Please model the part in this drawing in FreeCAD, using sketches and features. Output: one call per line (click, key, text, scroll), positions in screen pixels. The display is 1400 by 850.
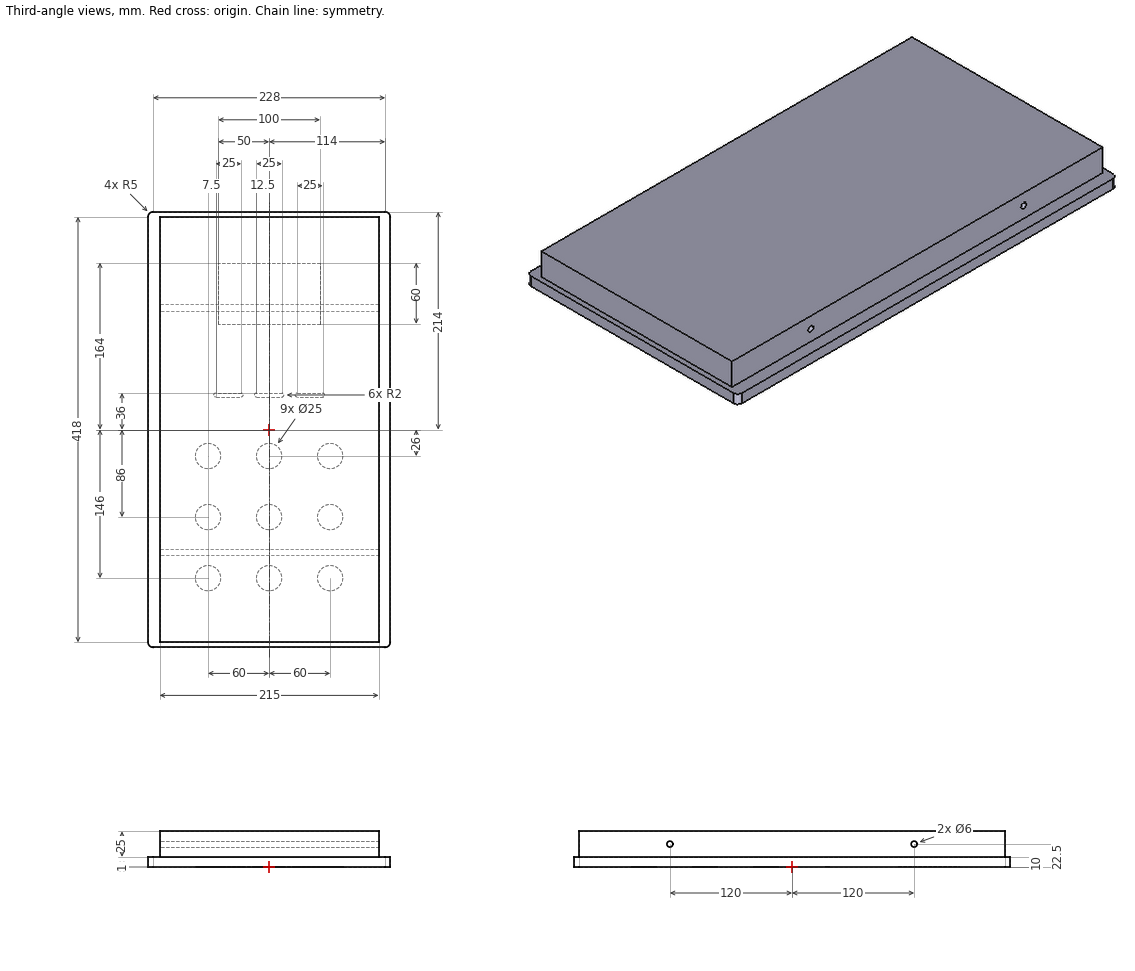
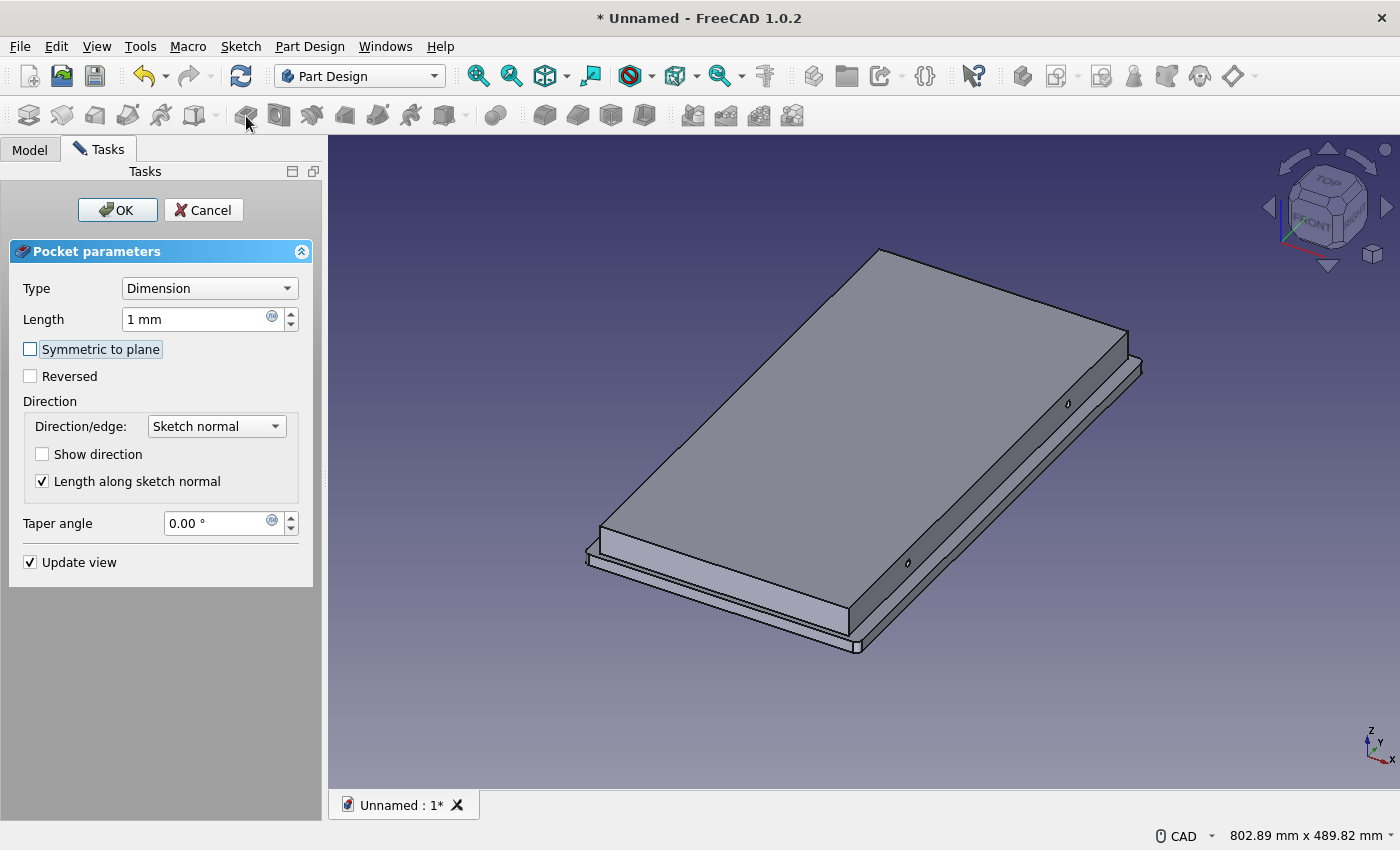
click(31, 376)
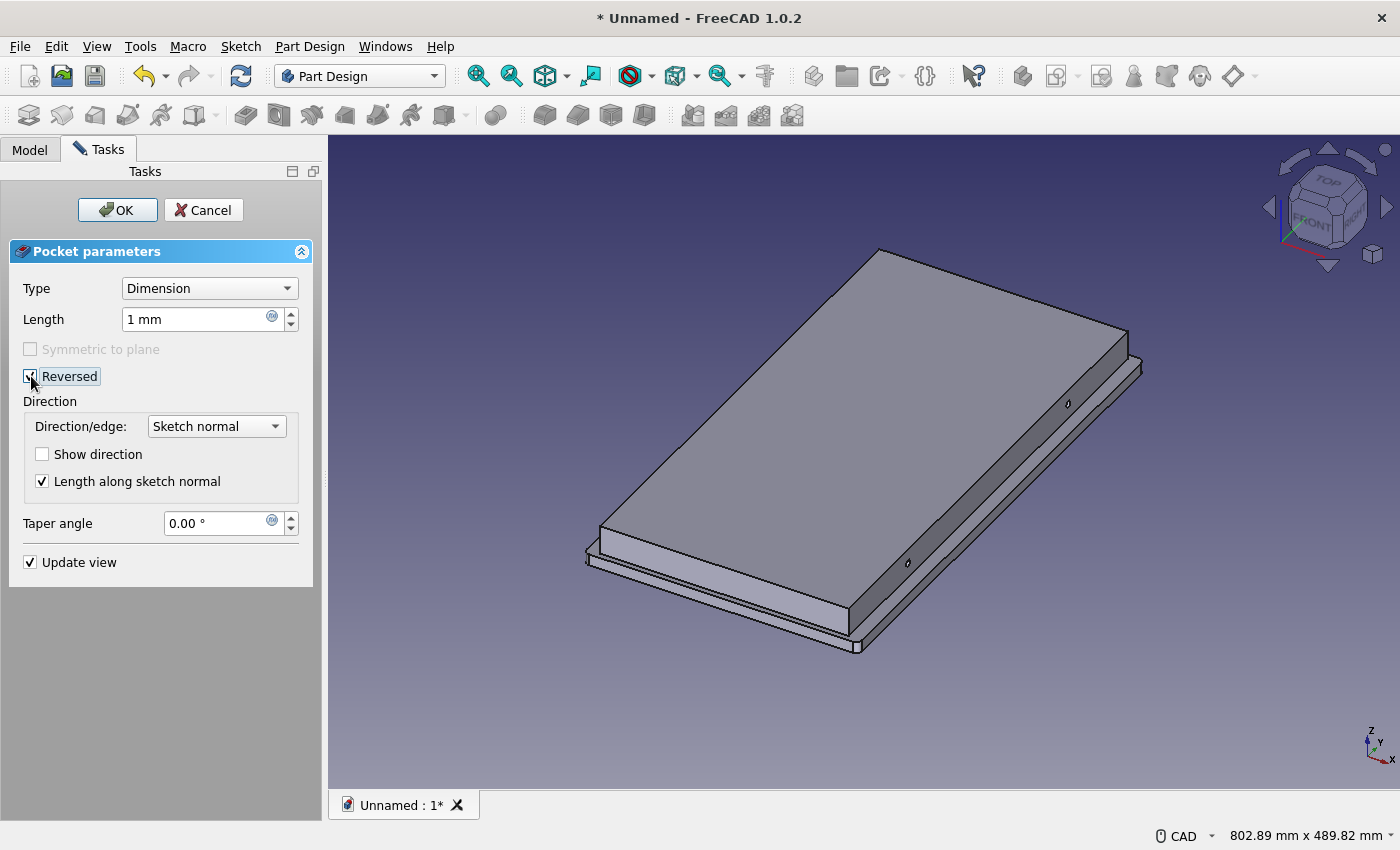
click(118, 210)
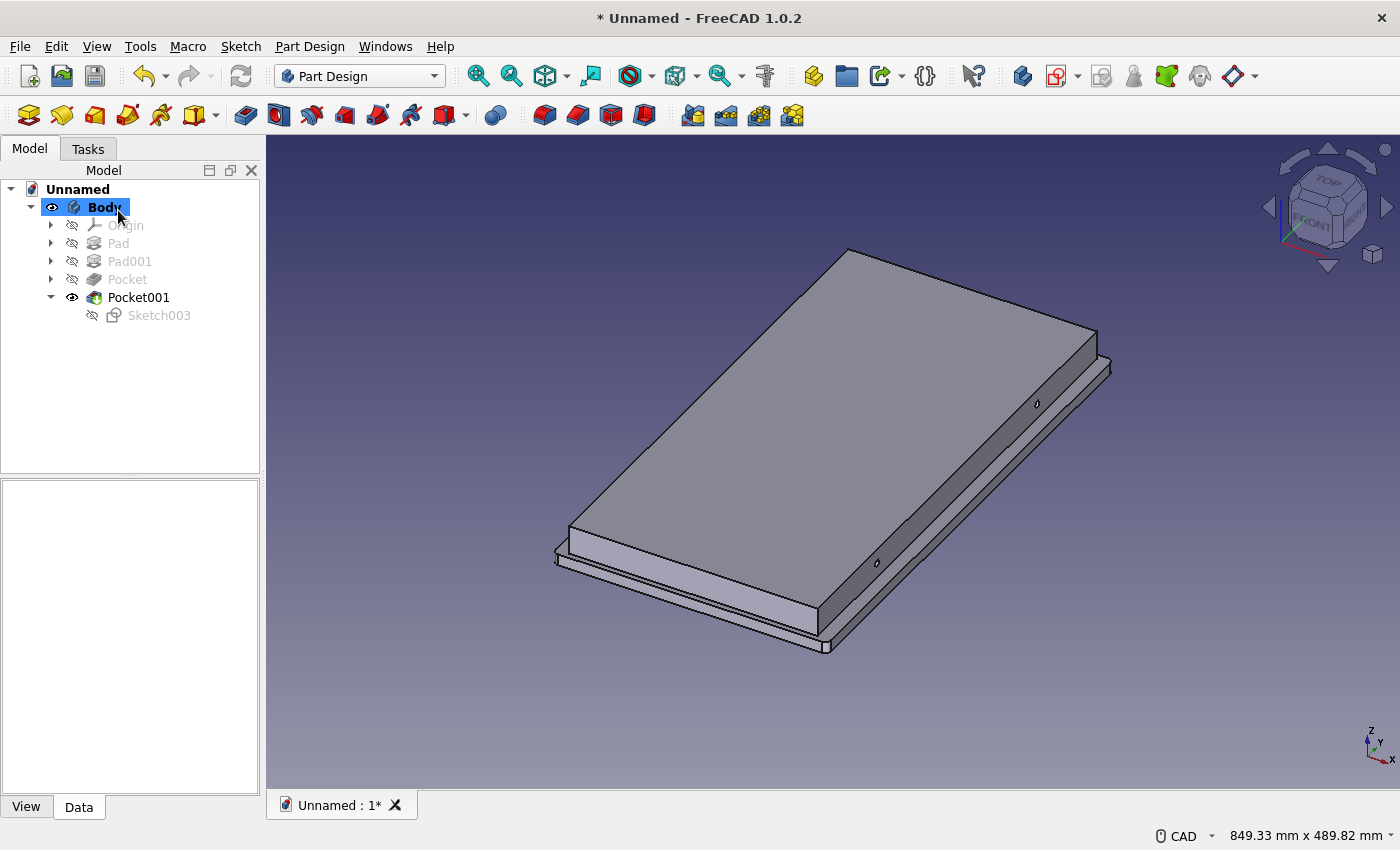
key(0)